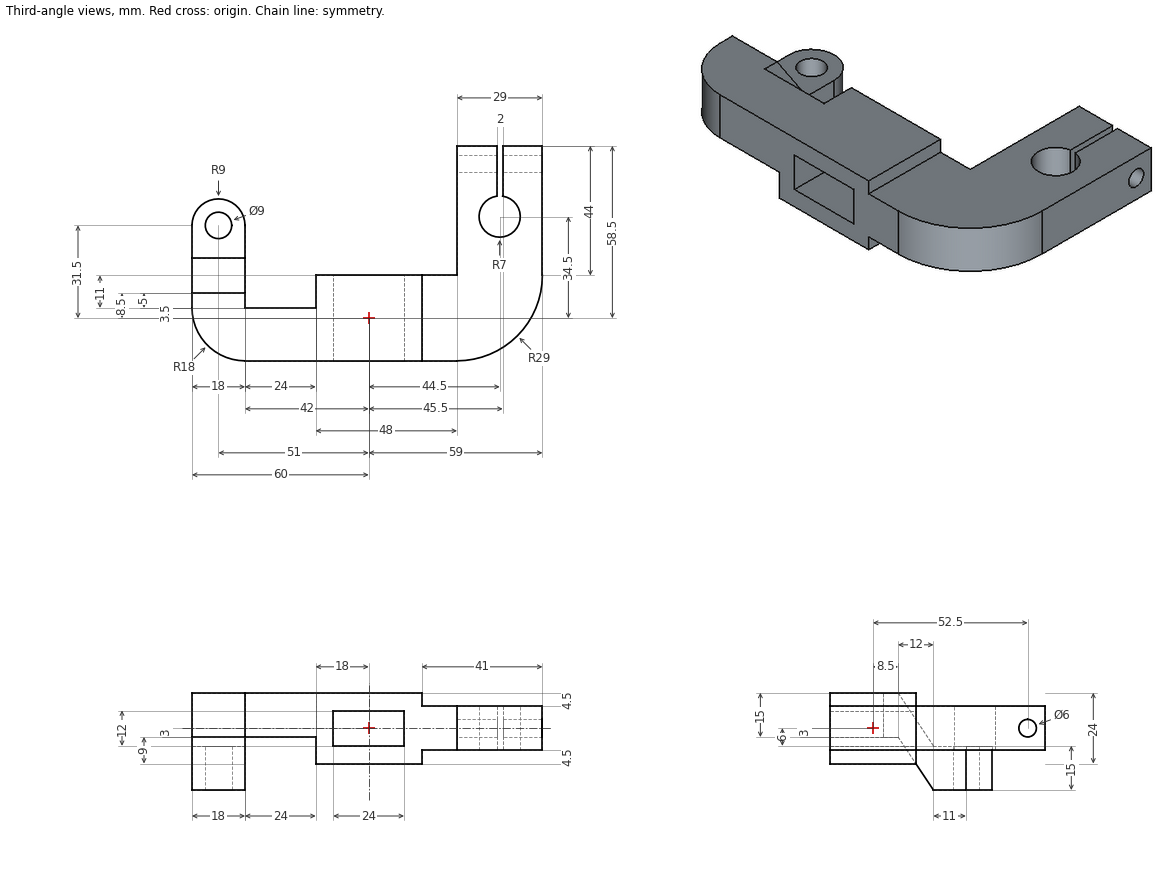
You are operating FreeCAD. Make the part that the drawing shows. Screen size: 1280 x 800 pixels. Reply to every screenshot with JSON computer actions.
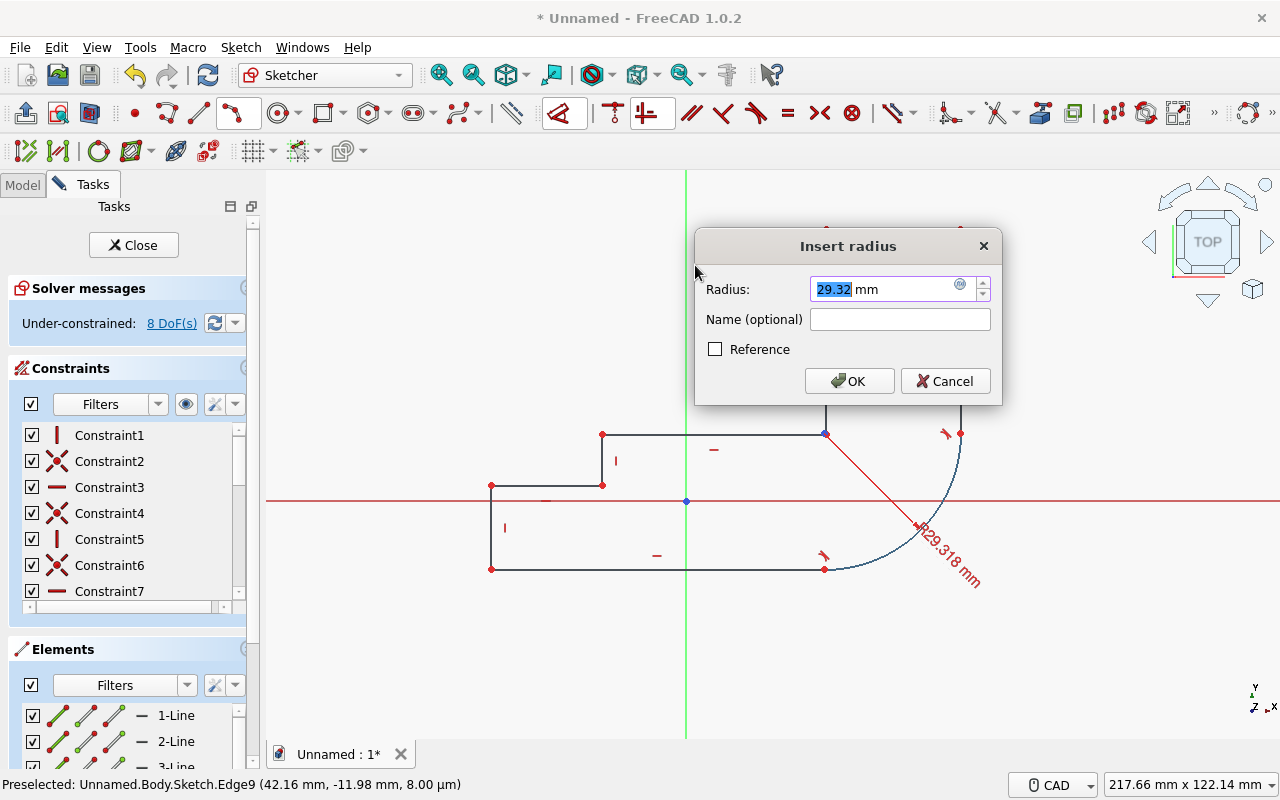
{"action": "type", "text": "29"}
{"action": "key", "text": "Return"}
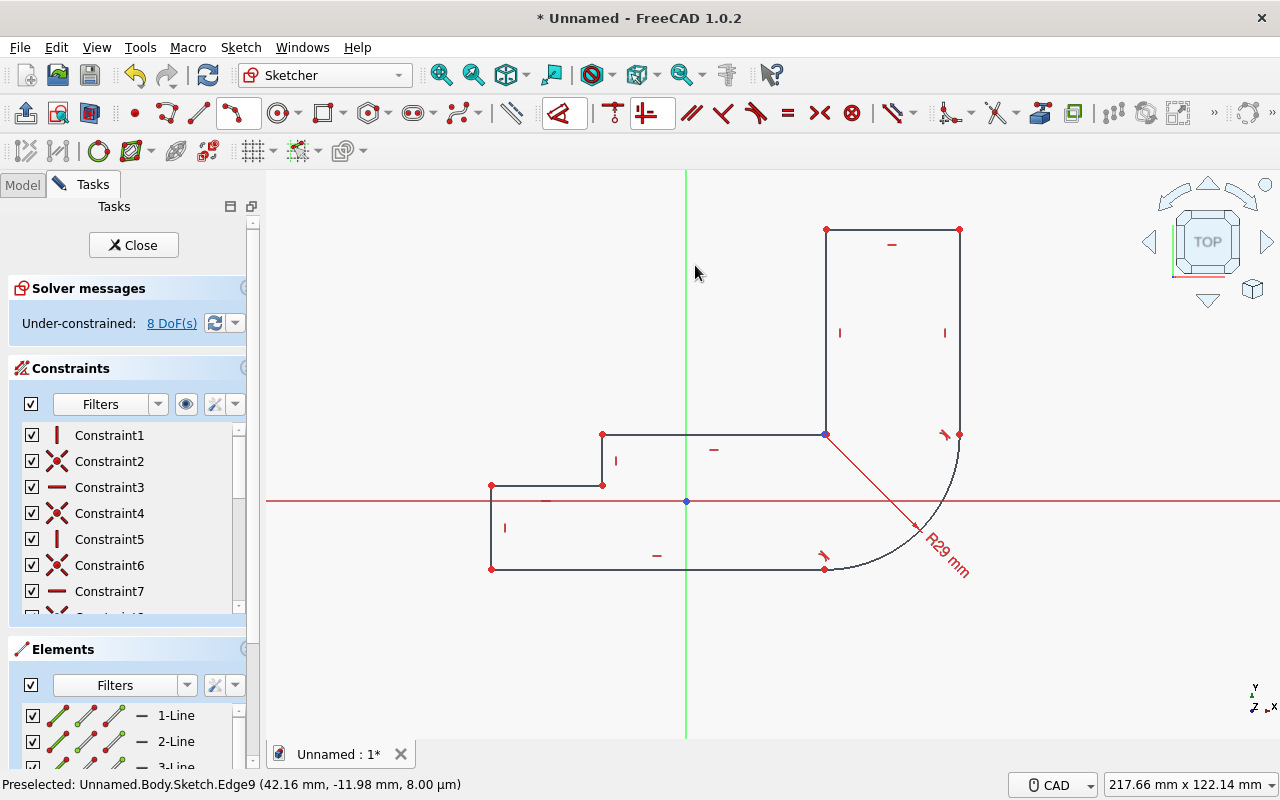
{"action": "left_click", "coordinate": [960, 373]}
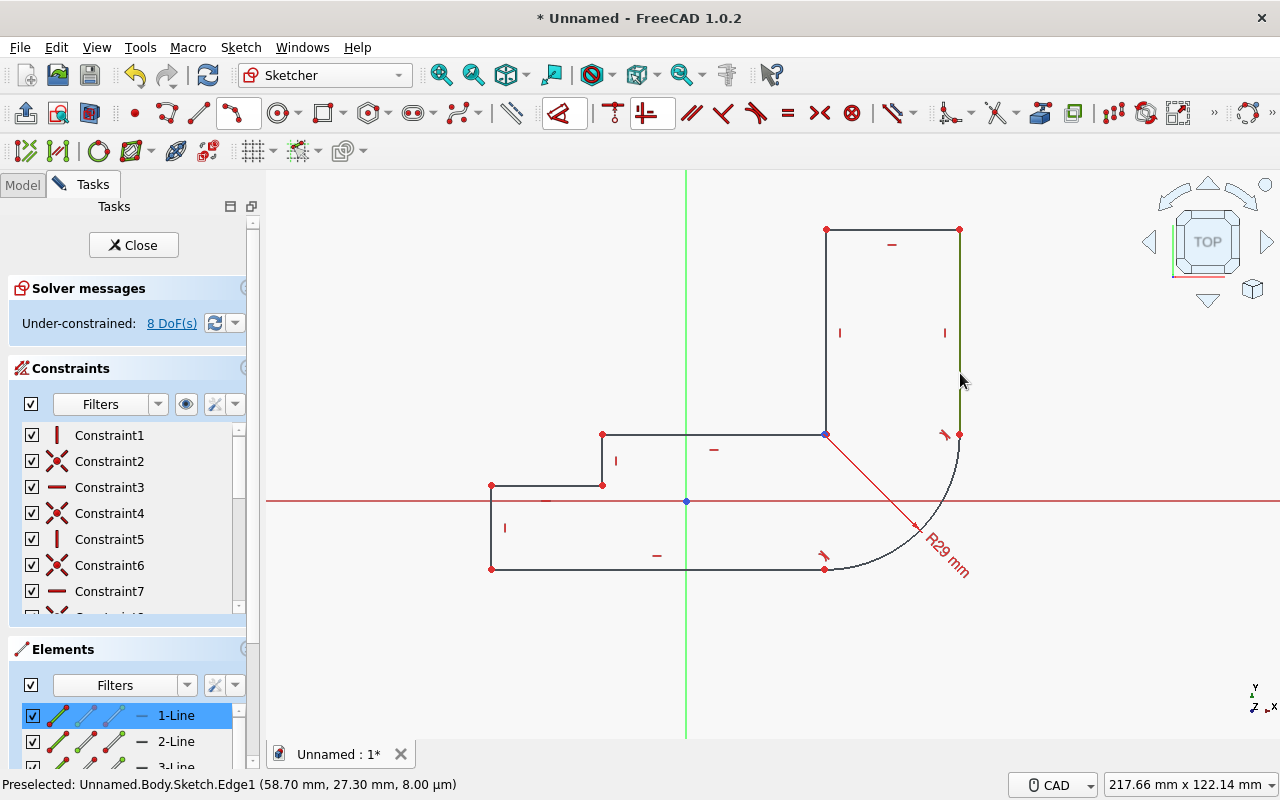
{"action": "left_click", "coordinate": [582, 114]}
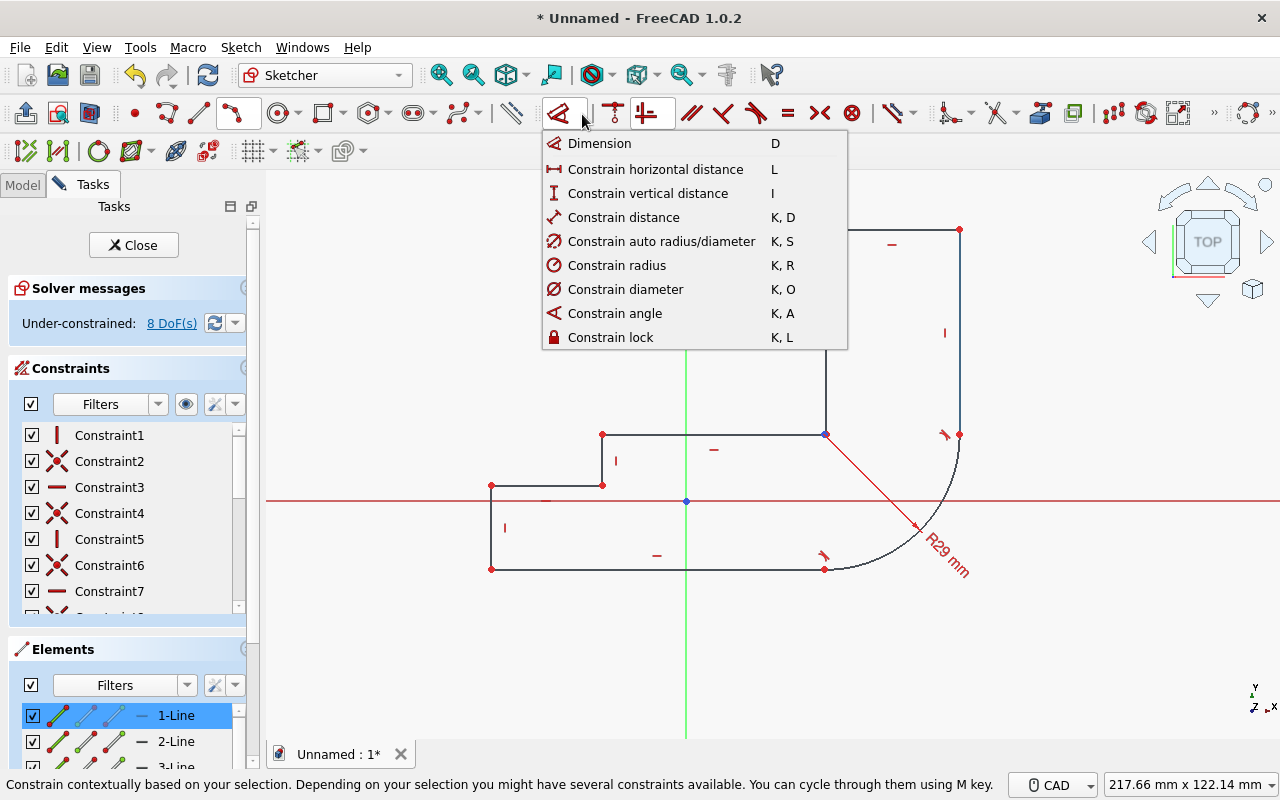
{"action": "left_click", "coordinate": [695, 193]}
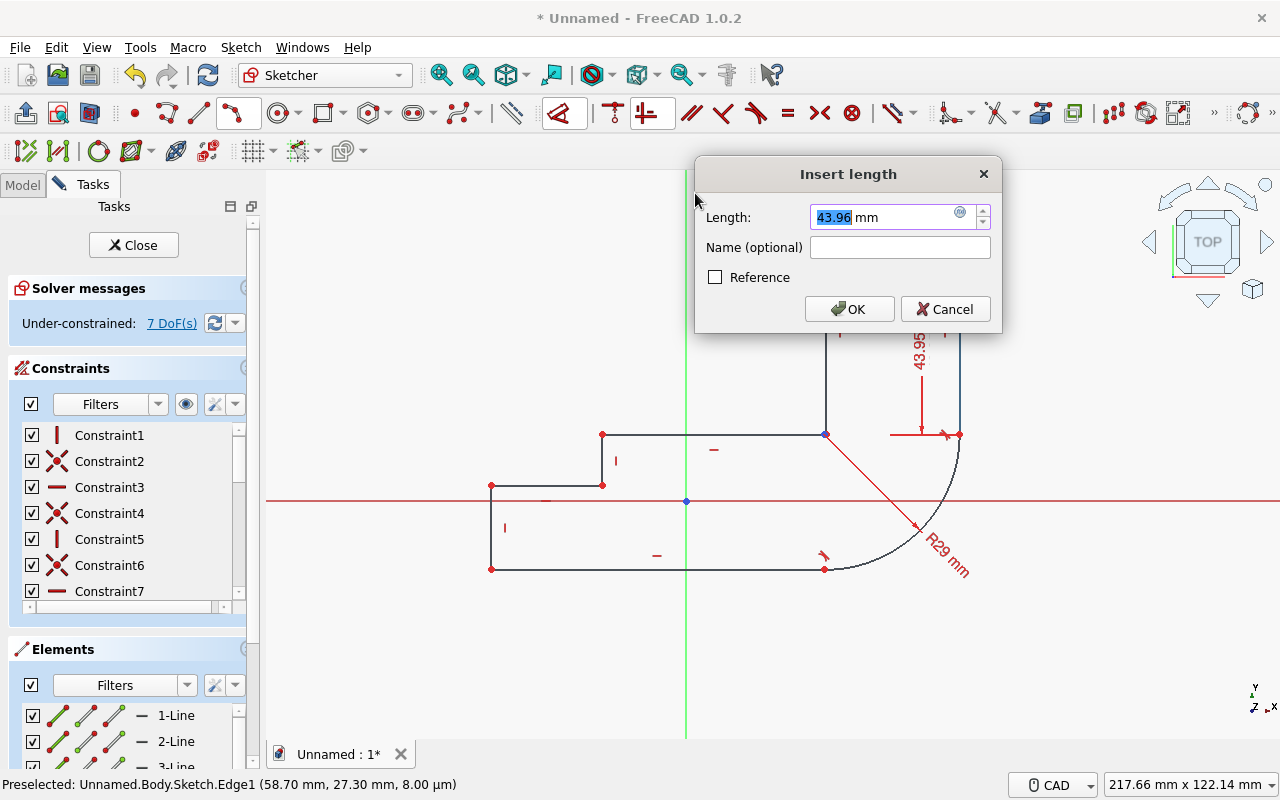
{"action": "type", "text": "44"}
{"action": "key", "text": "Return"}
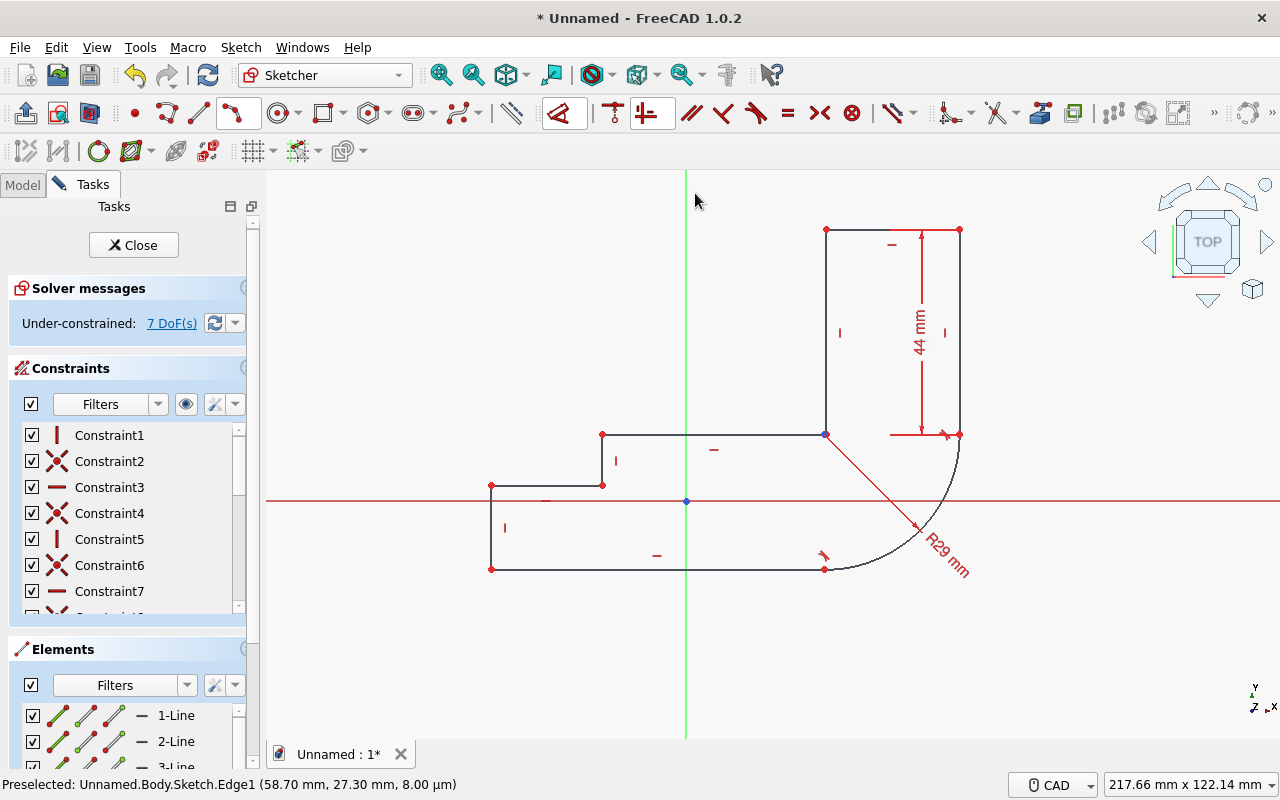
{"action": "left_click", "coordinate": [920, 230]}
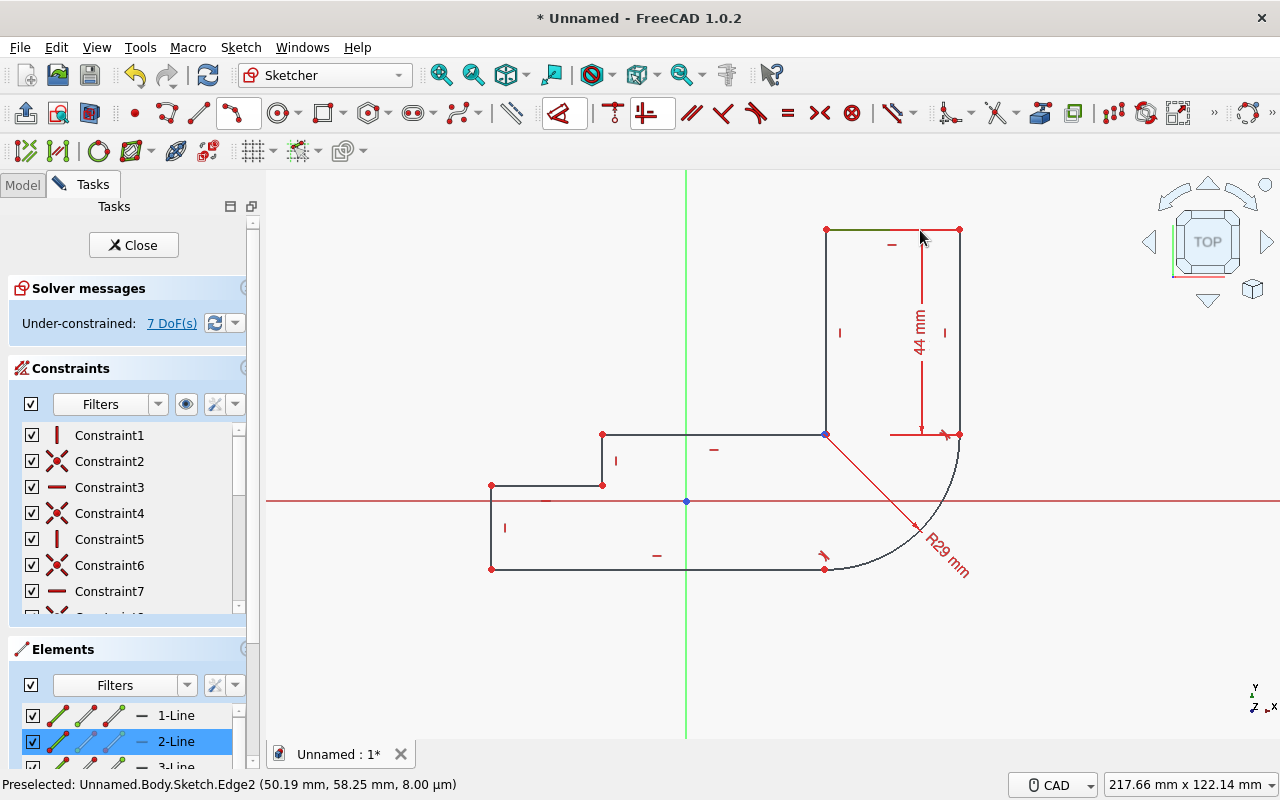
{"action": "left_click", "coordinate": [582, 114]}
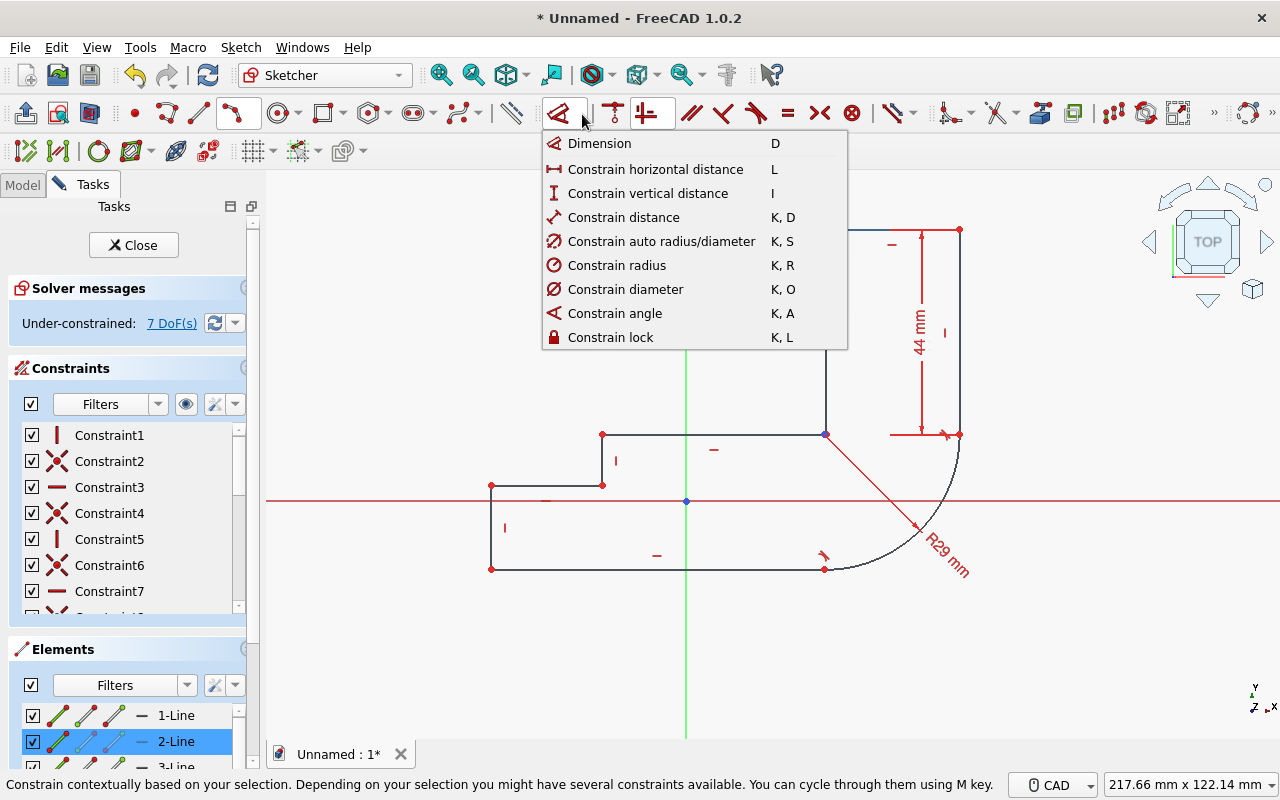
{"action": "left_click", "coordinate": [695, 169]}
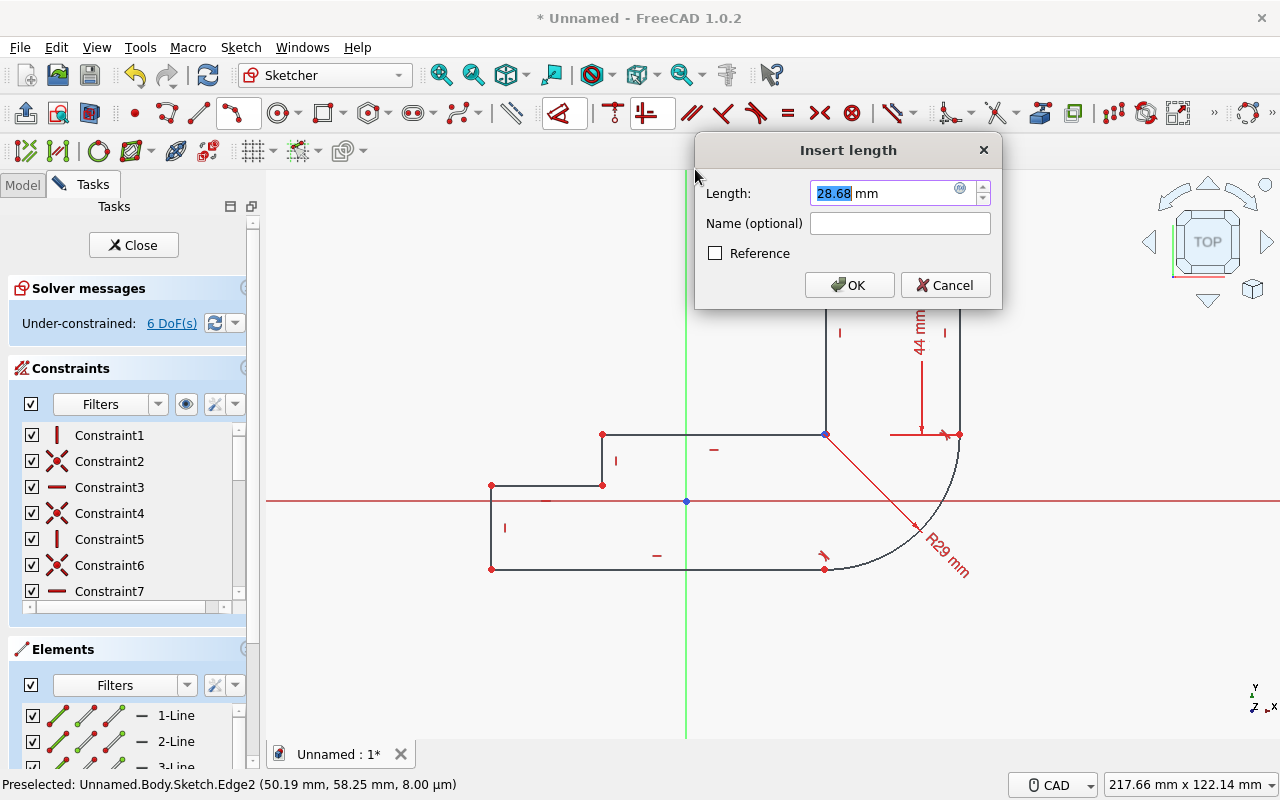
{"action": "type", "text": "29"}
{"action": "key", "text": "Return"}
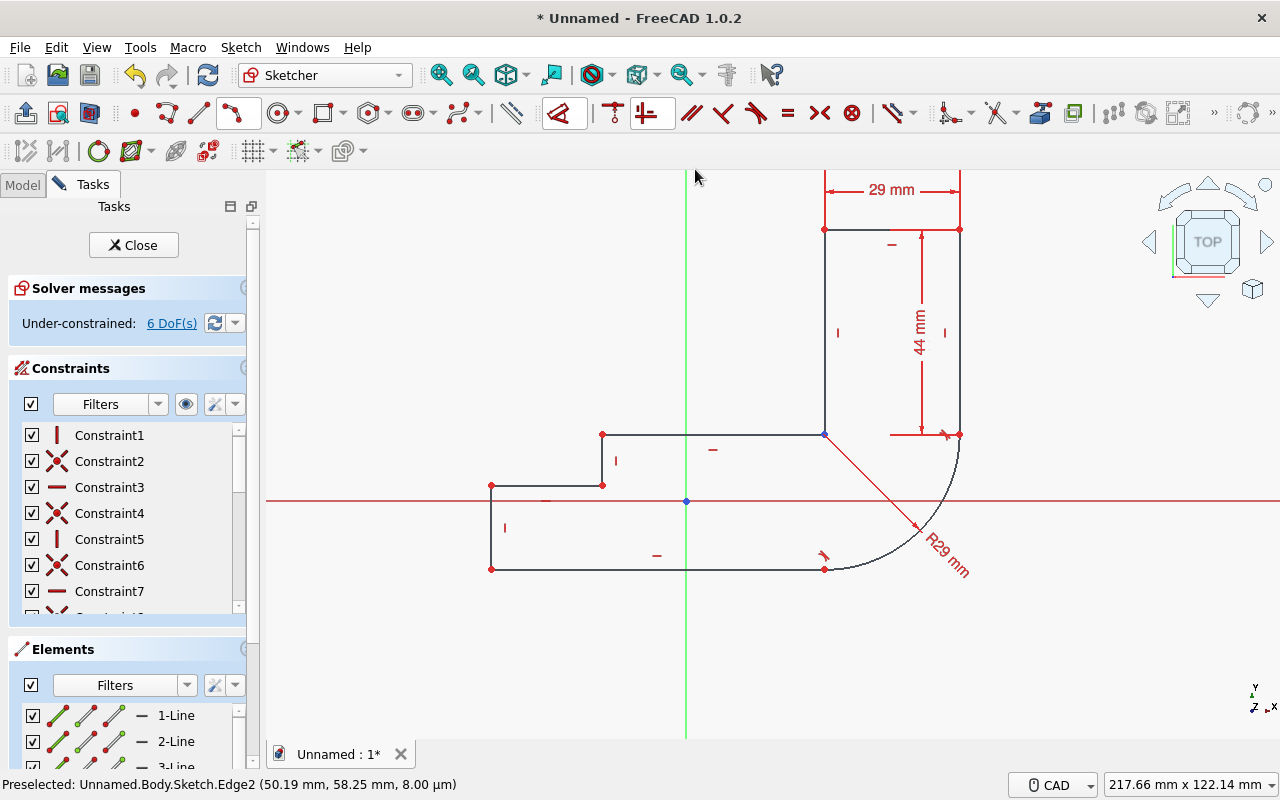
{"action": "left_click", "coordinate": [825, 291]}